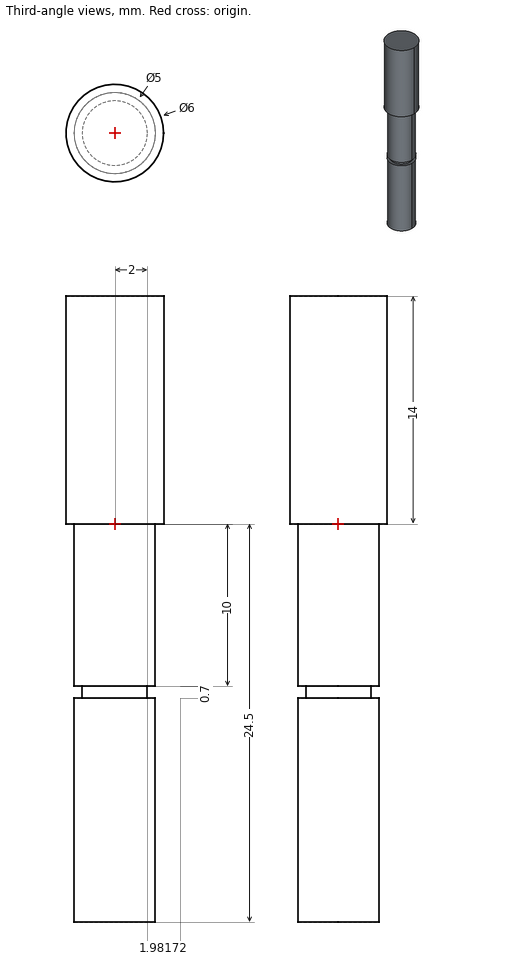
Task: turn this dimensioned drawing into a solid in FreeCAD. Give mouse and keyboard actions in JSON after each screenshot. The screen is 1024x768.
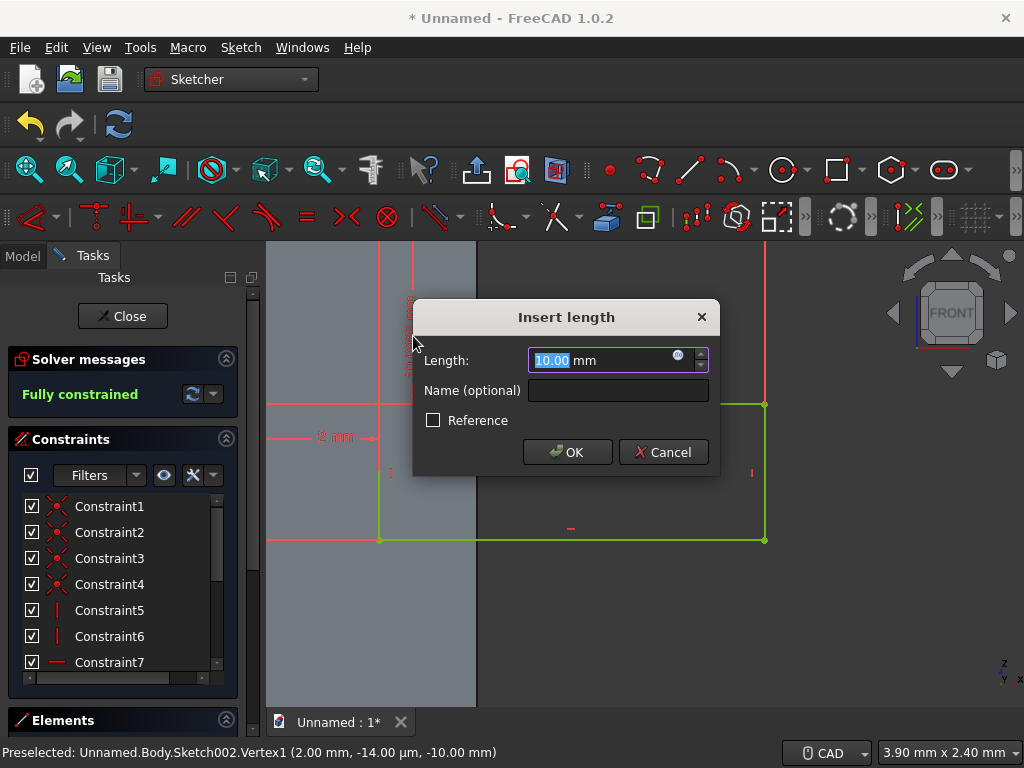
{"action": "type", "text": "10"}
{"action": "key", "text": "Return"}
{"action": "key", "text": "Escape"}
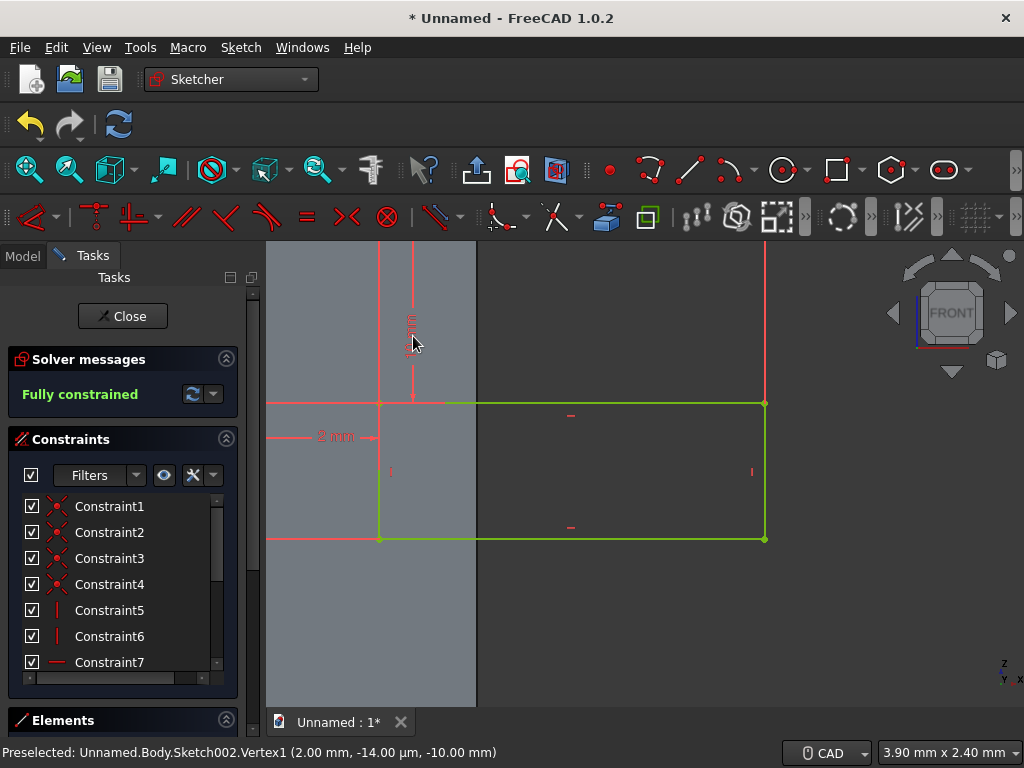
{"action": "left_click", "coordinate": [123, 316]}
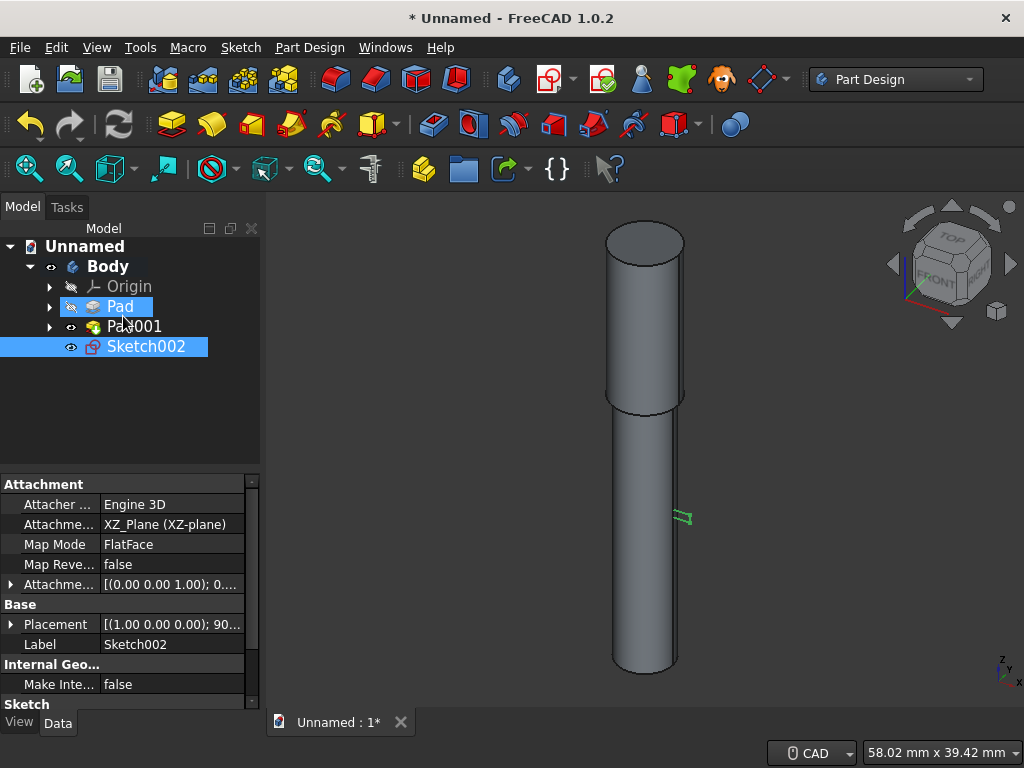
{"action": "left_click", "coordinate": [514, 124]}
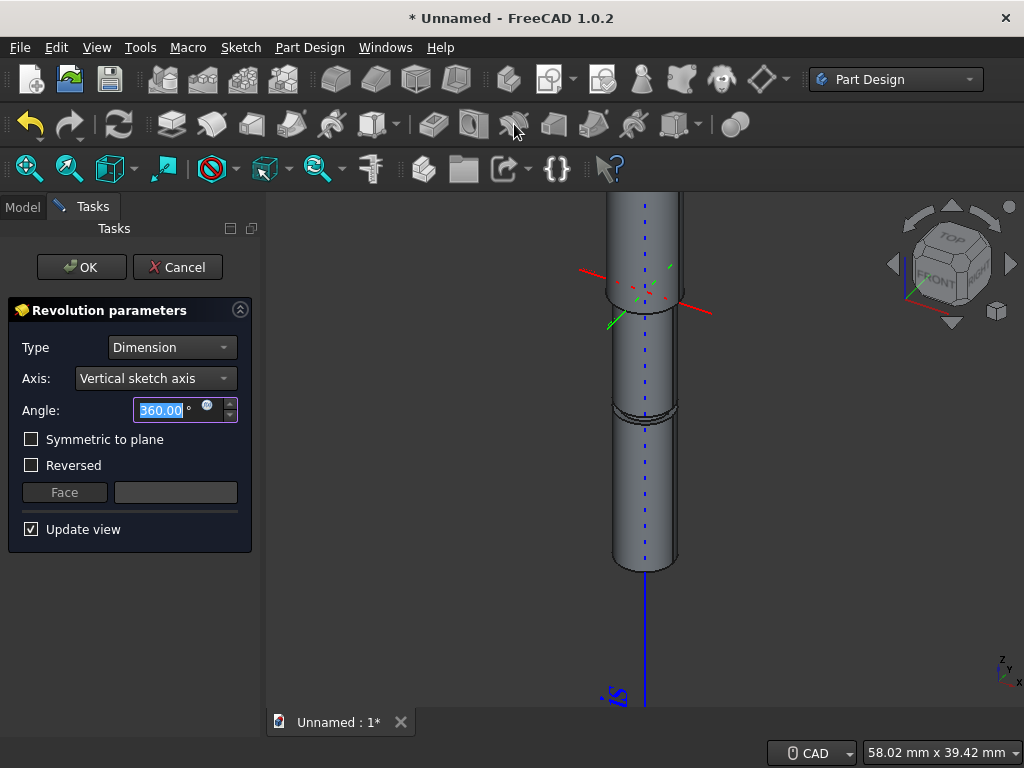
{"action": "left_click", "coordinate": [82, 267]}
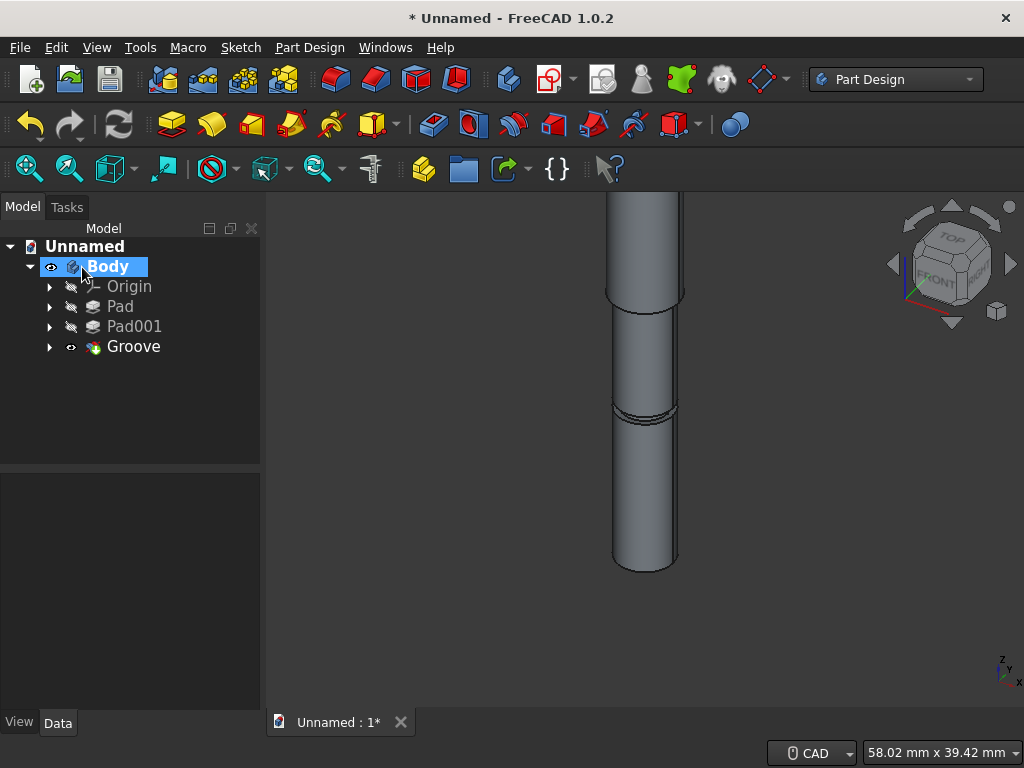
{"action": "key", "text": "0"}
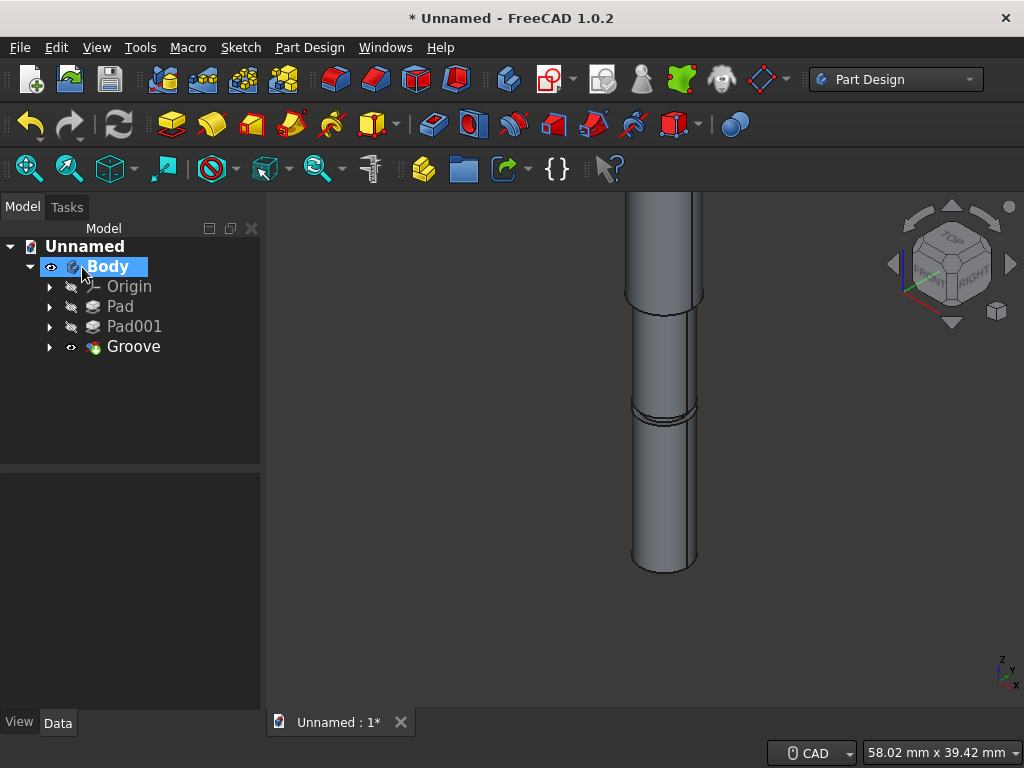
{"action": "left_click", "coordinate": [30, 170]}